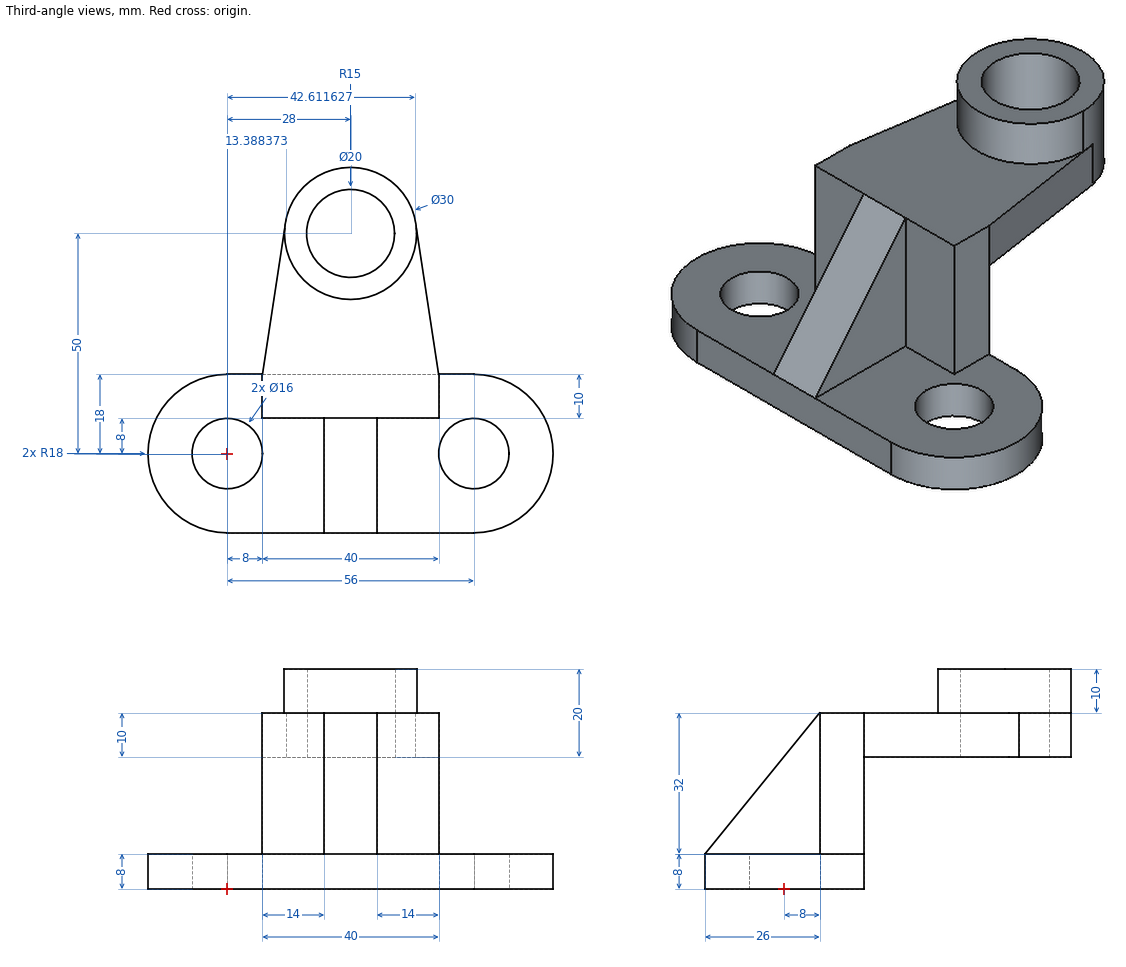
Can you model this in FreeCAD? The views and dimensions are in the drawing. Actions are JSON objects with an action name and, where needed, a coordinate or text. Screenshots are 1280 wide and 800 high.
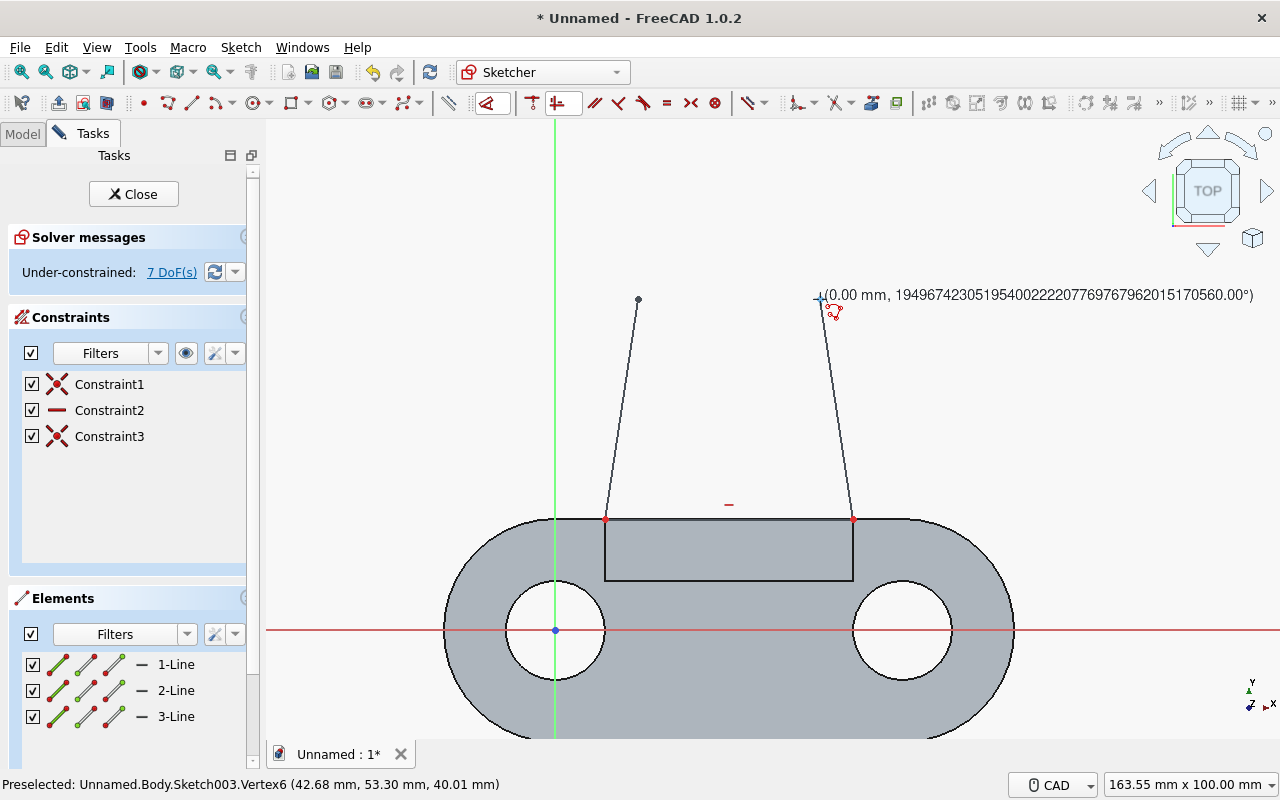
{"action": "key", "text": "g 3 a"}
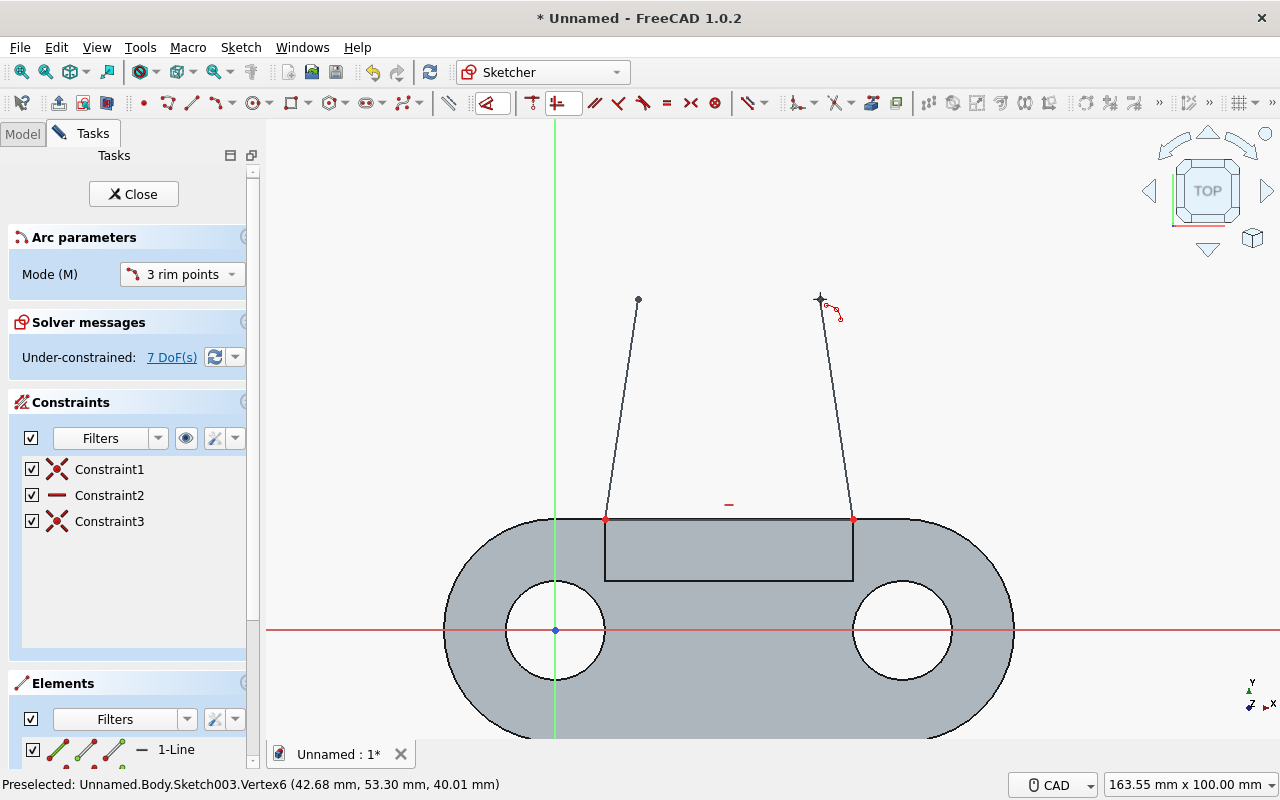
{"action": "left_click", "coordinate": [820, 300]}
{"action": "left_click", "coordinate": [638, 300]}
{"action": "left_click", "coordinate": [729, 227]}
{"action": "key", "text": "Escape"}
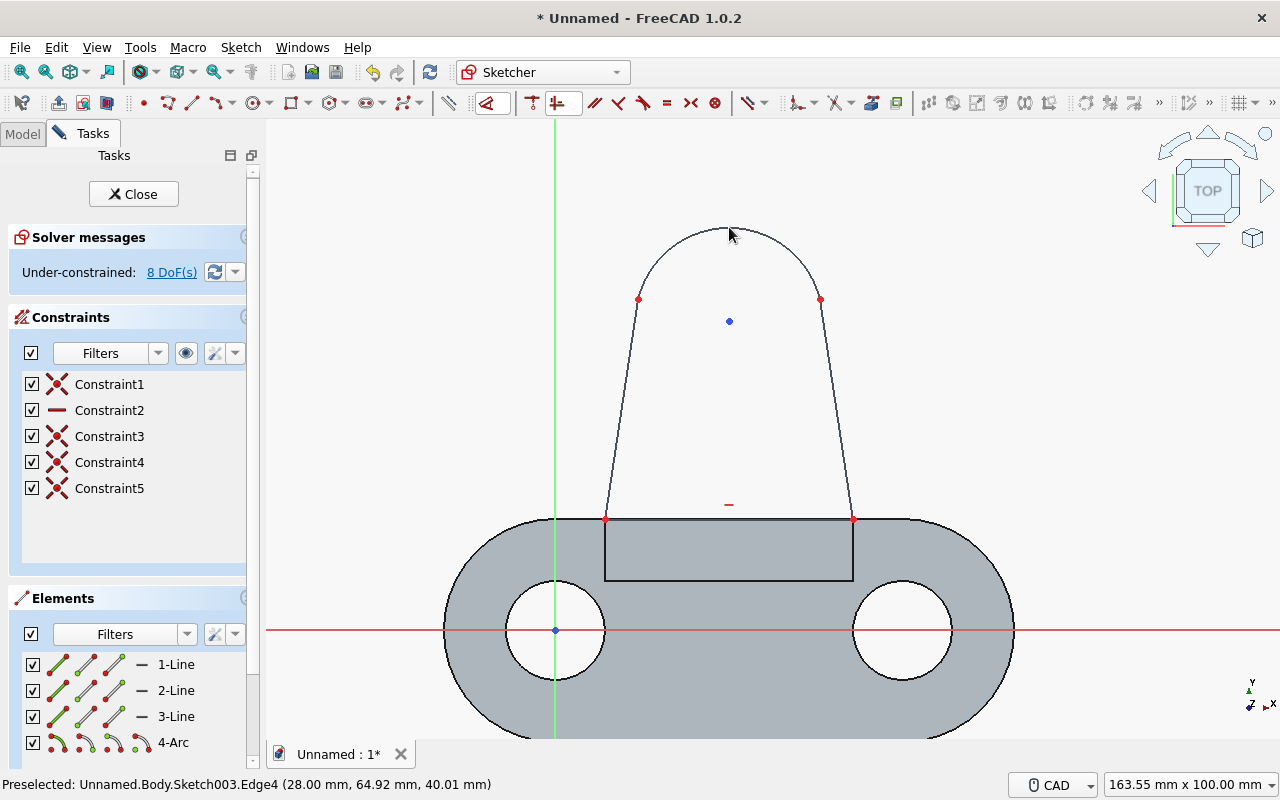
{"action": "left_click", "coordinate": [777, 241]}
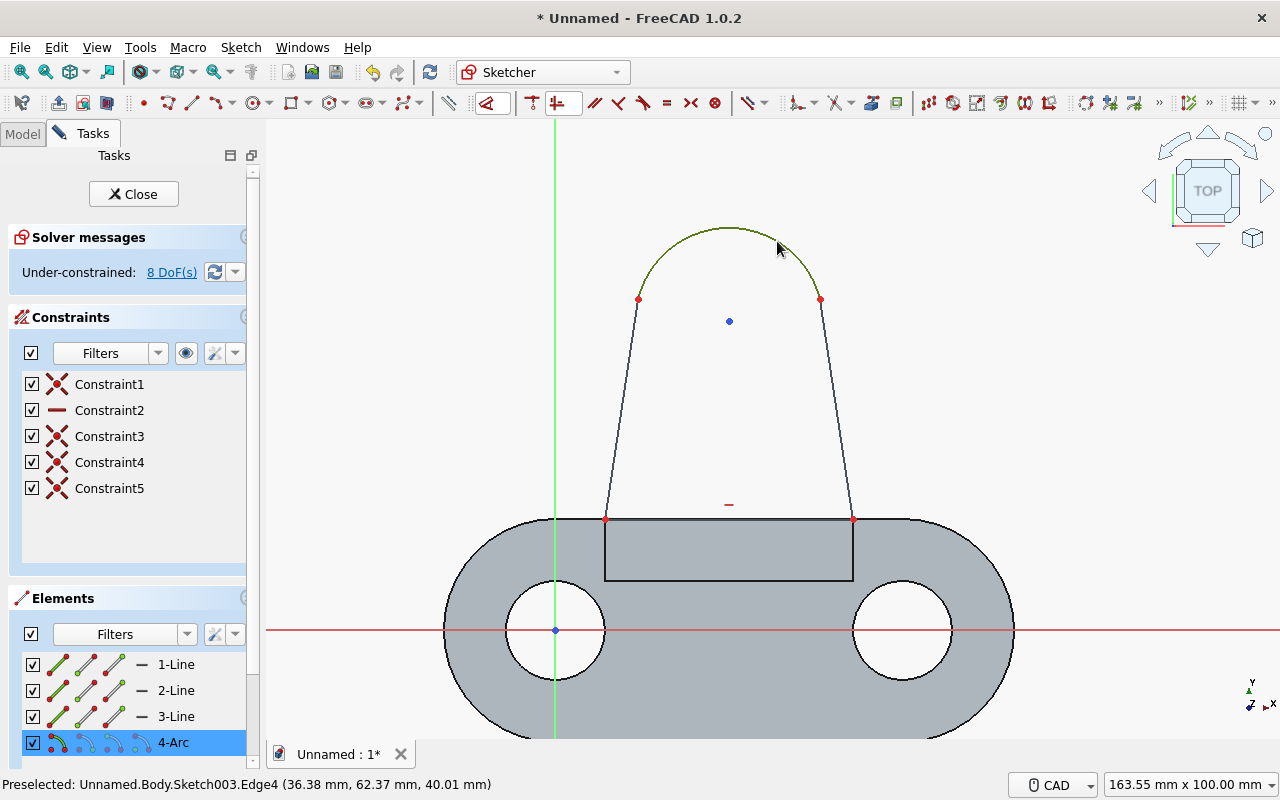
{"action": "key", "text": "k r"}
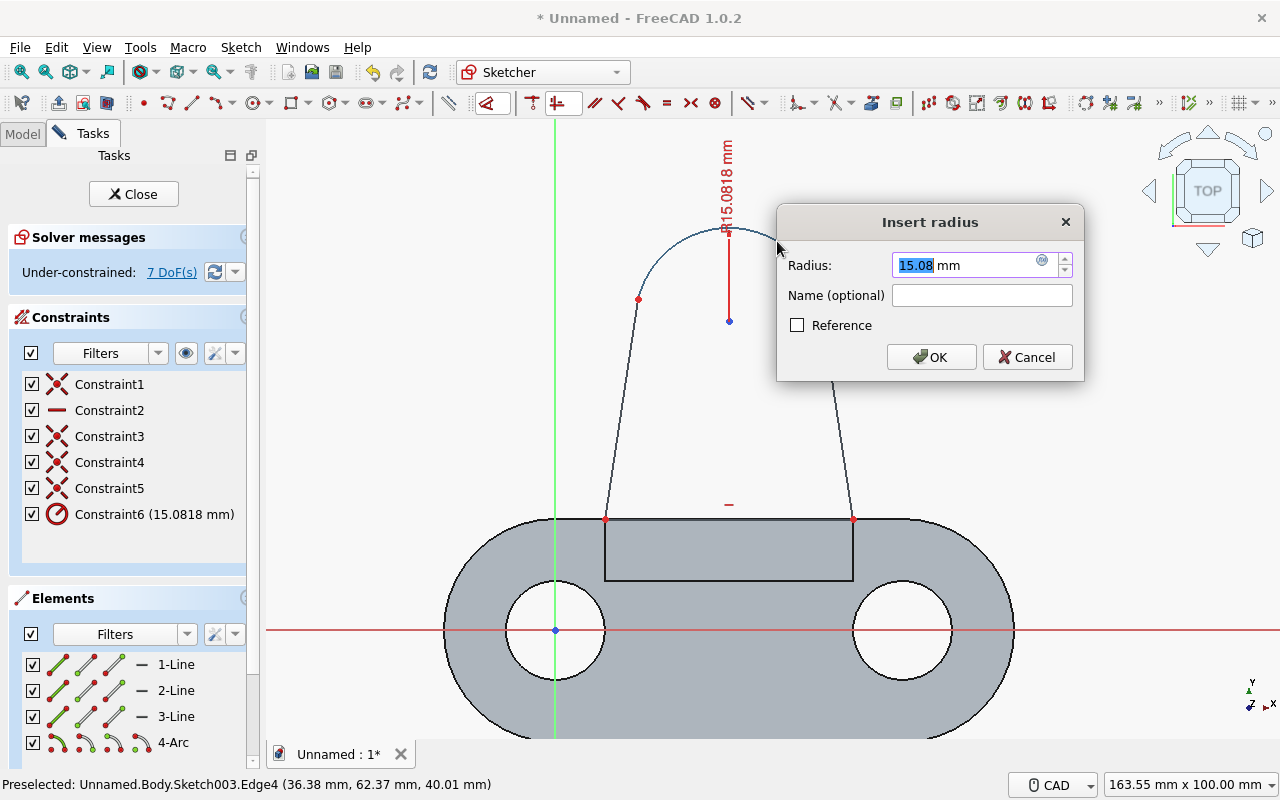
{"action": "type", "text": "15"}
{"action": "key", "text": "Return"}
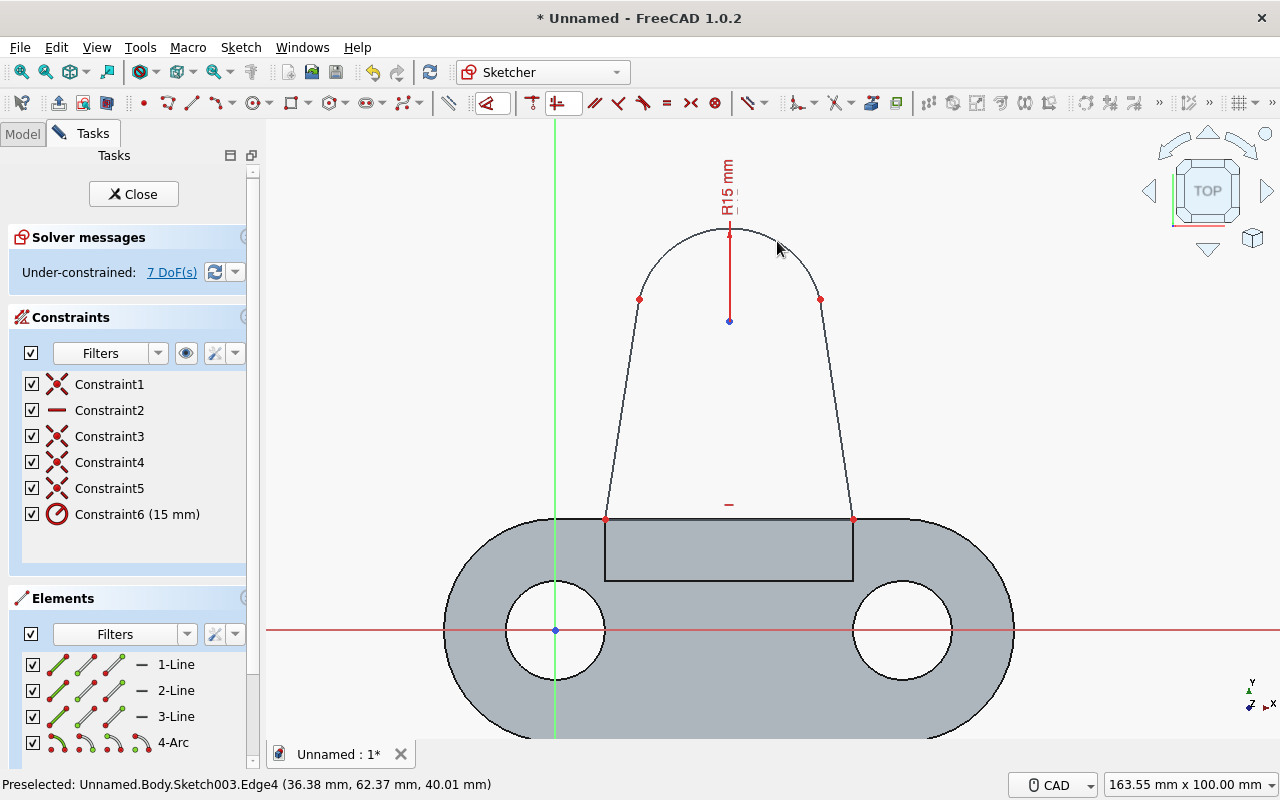
{"action": "left_click", "coordinate": [679, 520]}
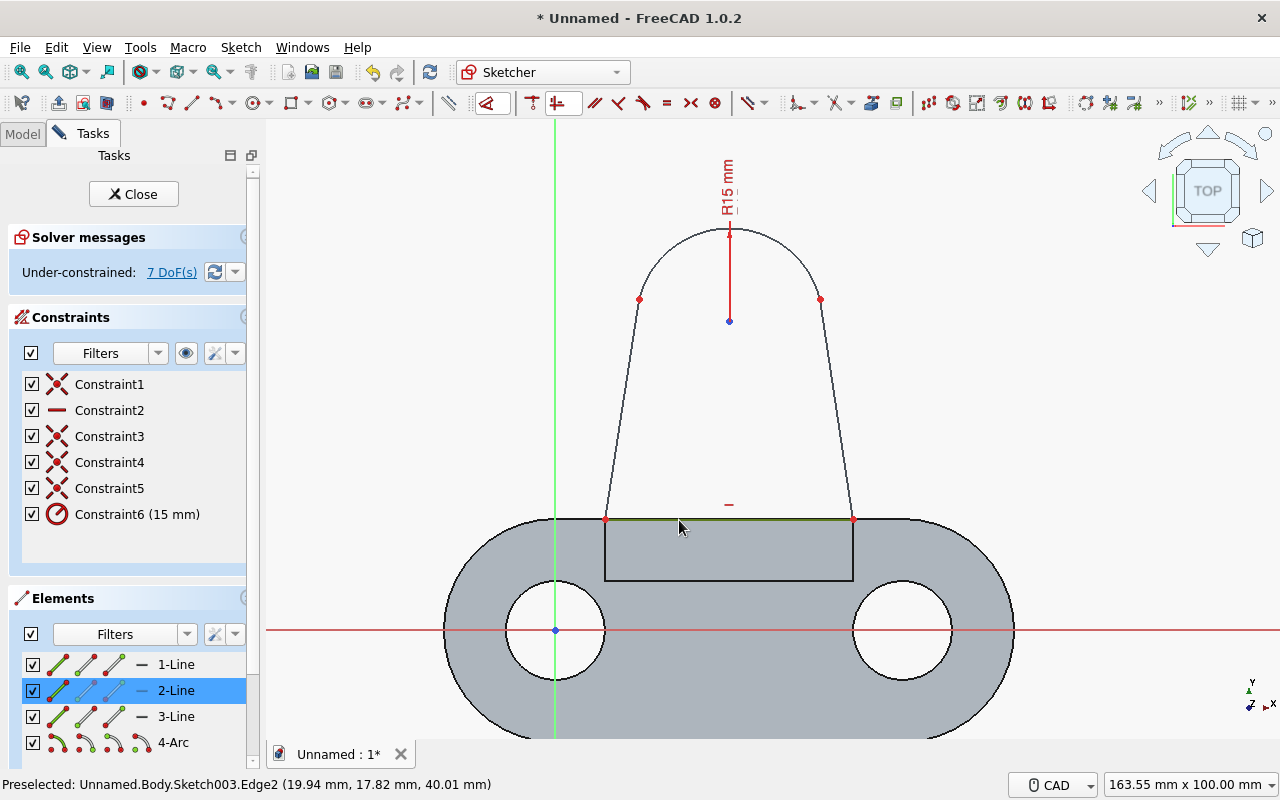
{"action": "left_click", "coordinate": [504, 104]}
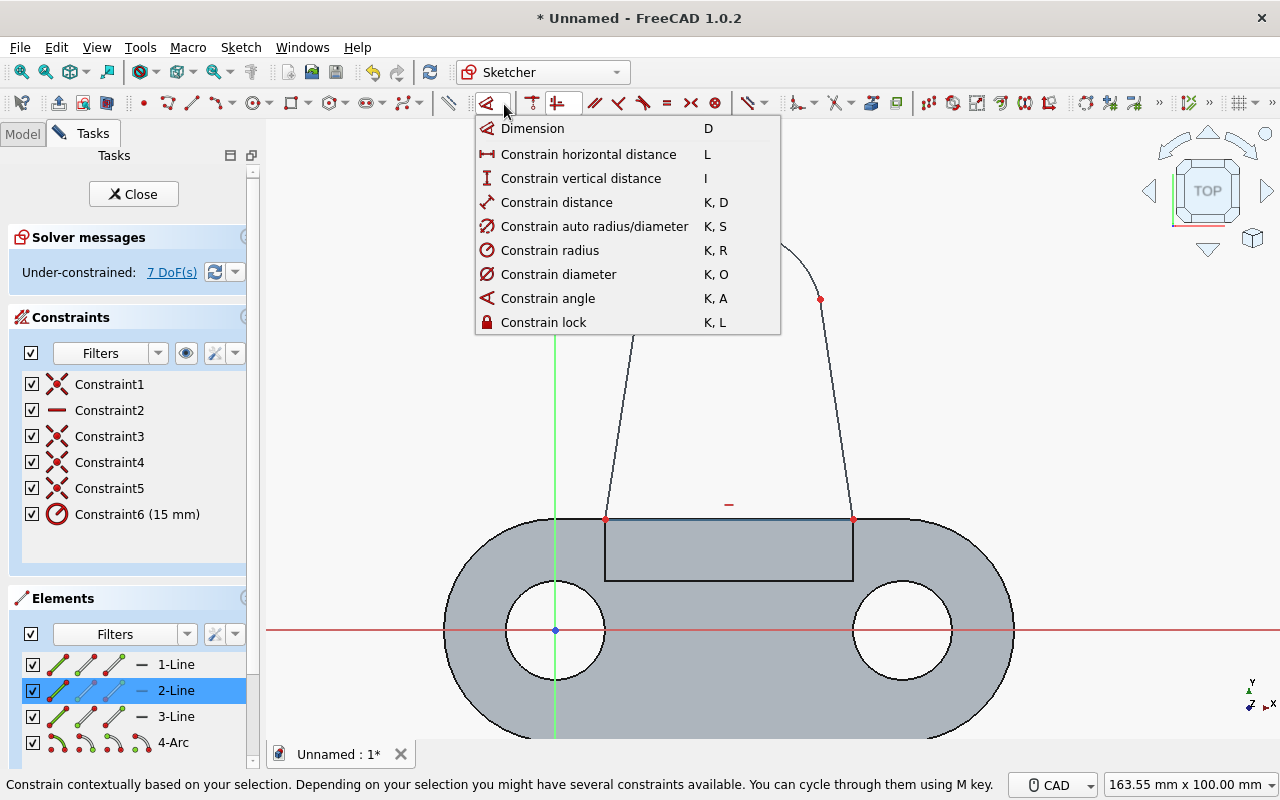
{"action": "left_click", "coordinate": [628, 154]}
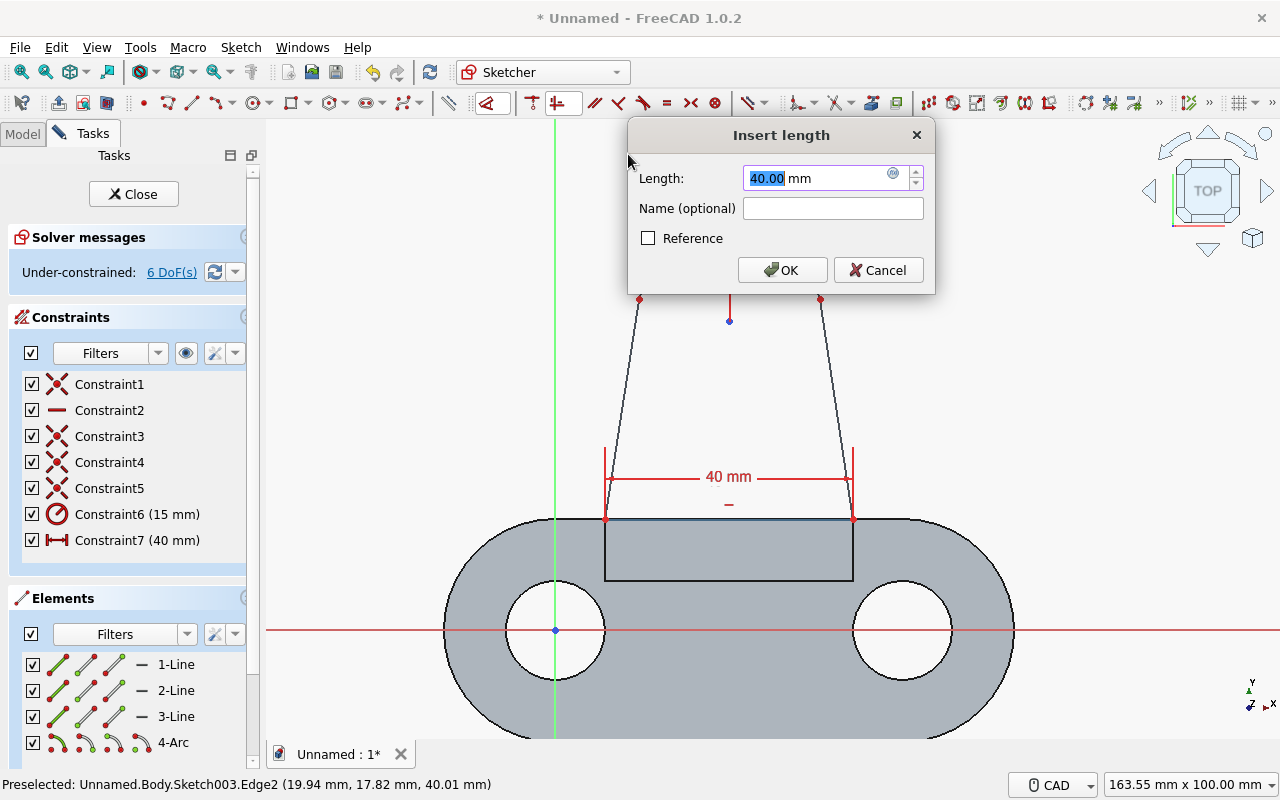
{"action": "type", "text": "40"}
{"action": "key", "text": "Return"}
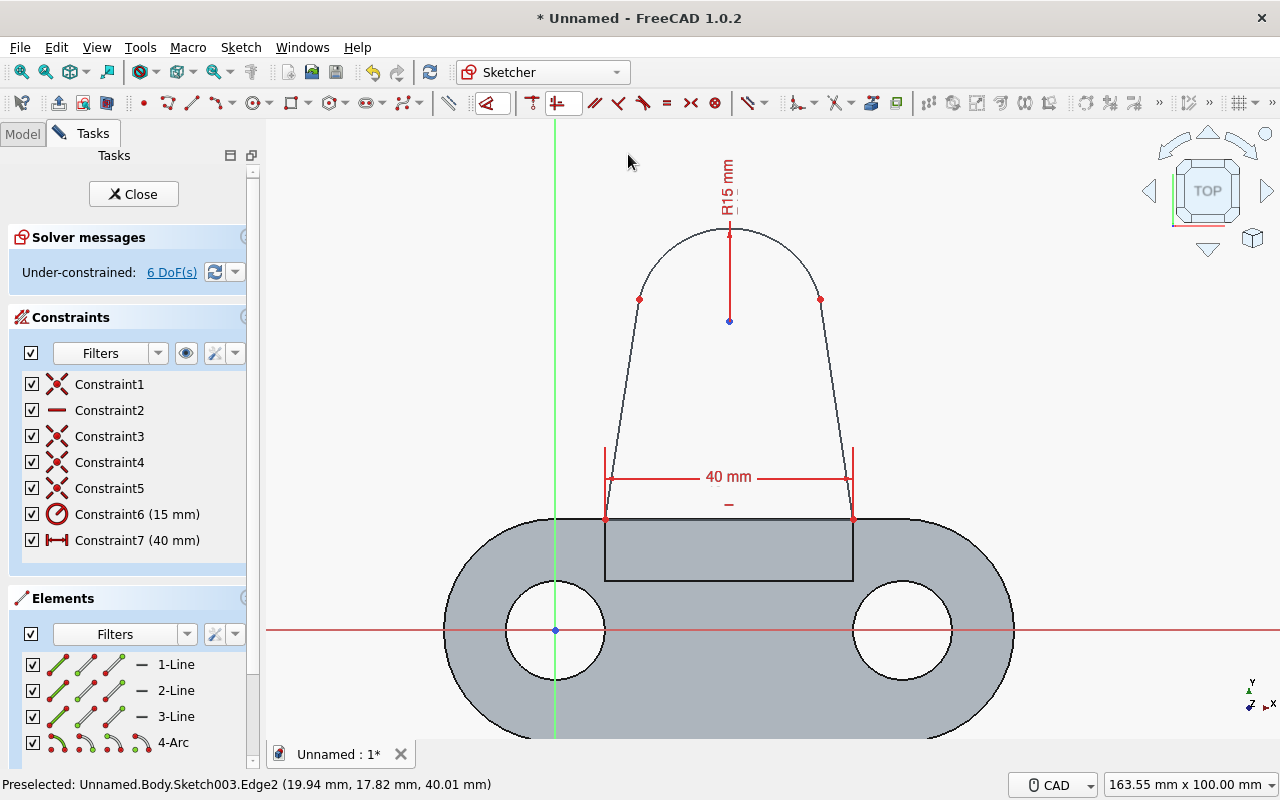
{"action": "left_click", "coordinate": [605, 520]}